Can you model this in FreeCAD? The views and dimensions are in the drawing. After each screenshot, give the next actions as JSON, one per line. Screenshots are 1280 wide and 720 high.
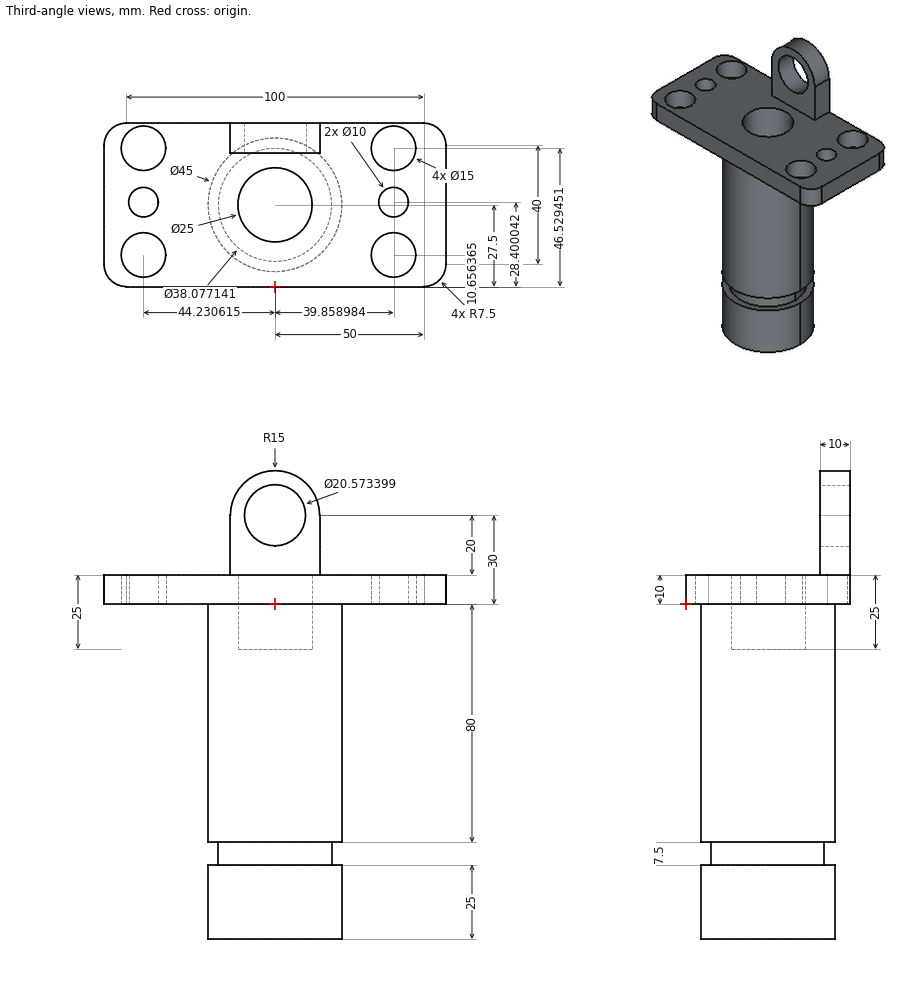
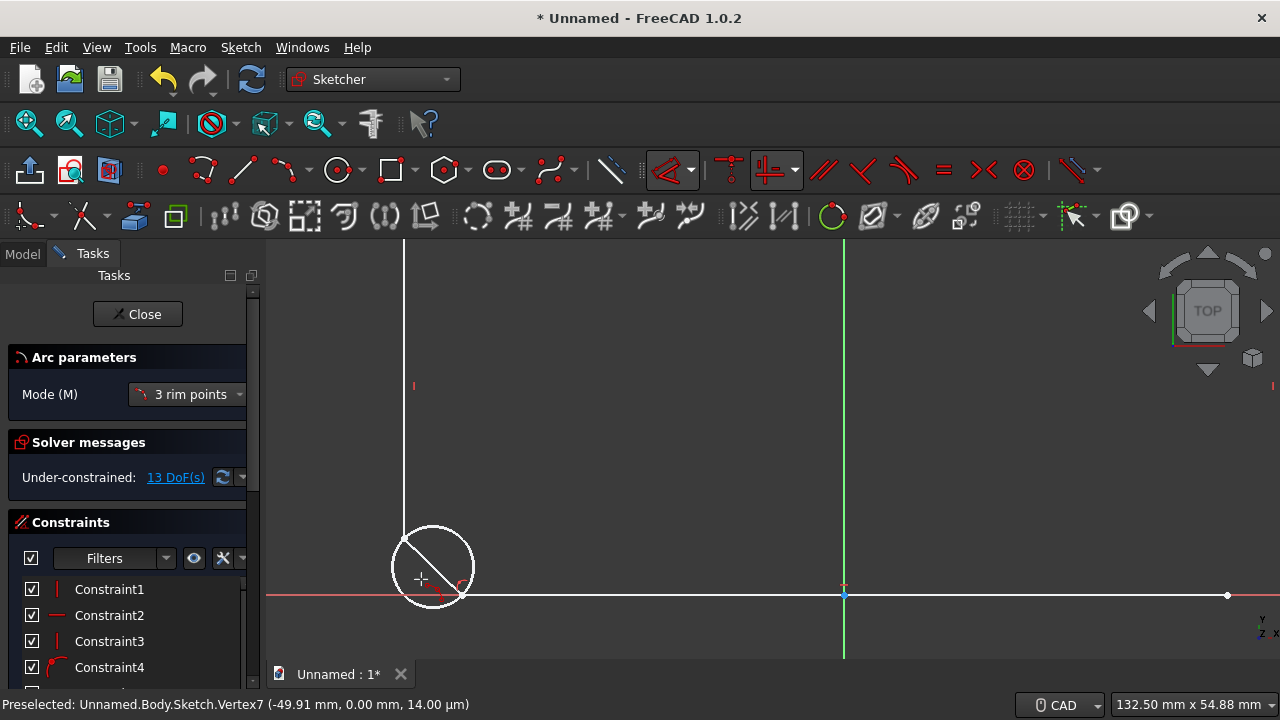
{"action": "left_click", "coordinate": [421, 579]}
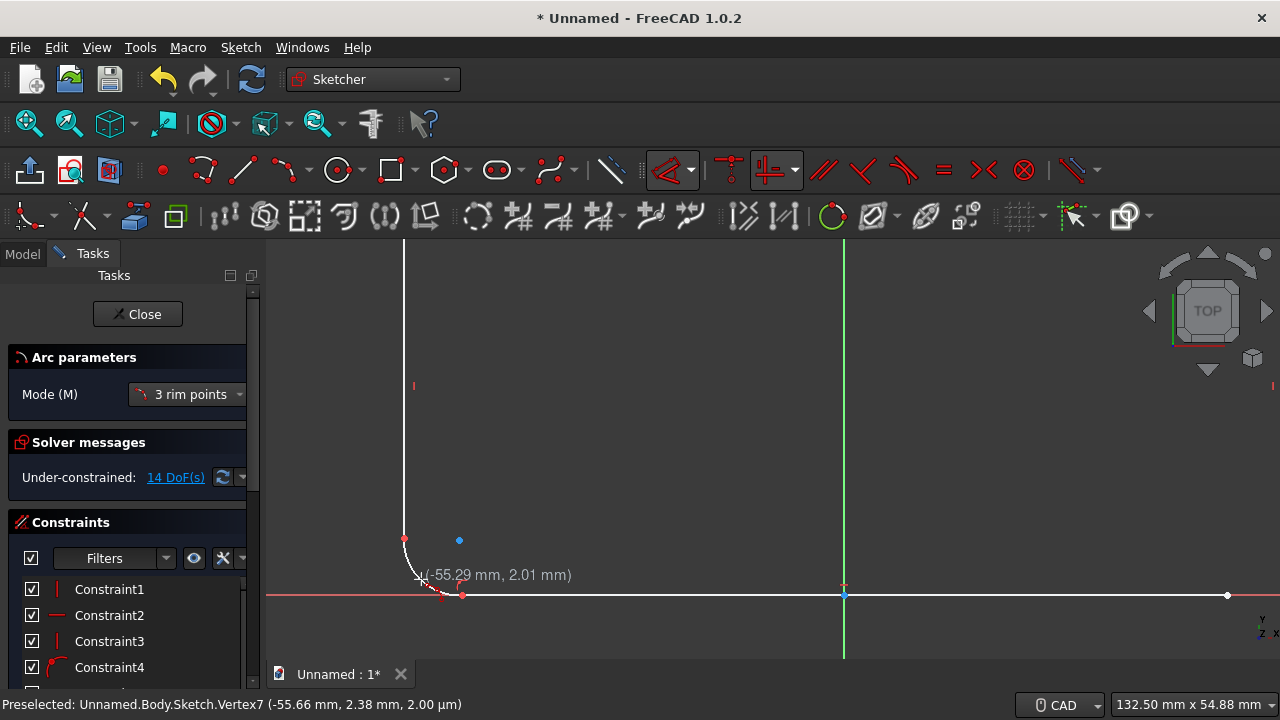
{"action": "scroll", "coordinate": [421, 579], "scroll_direction": "down", "scroll_amount": 2}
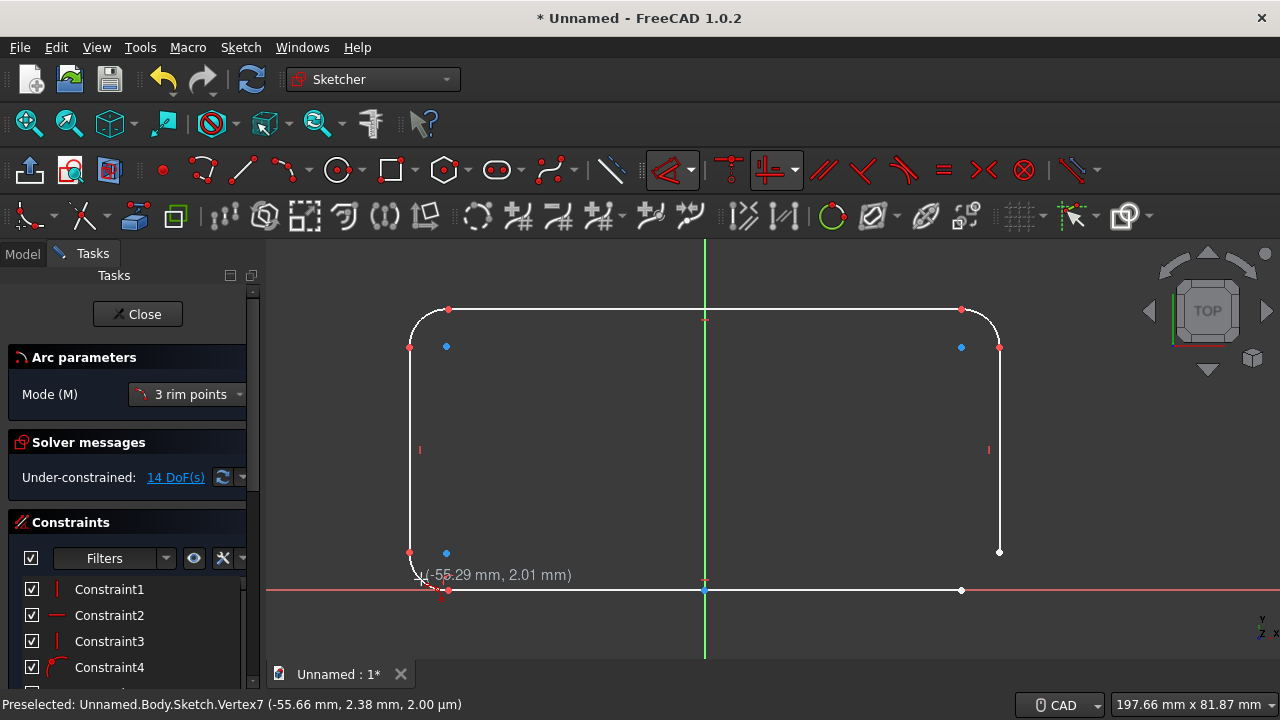
{"action": "left_click", "coordinate": [962, 590]}
{"action": "left_click", "coordinate": [1000, 552]}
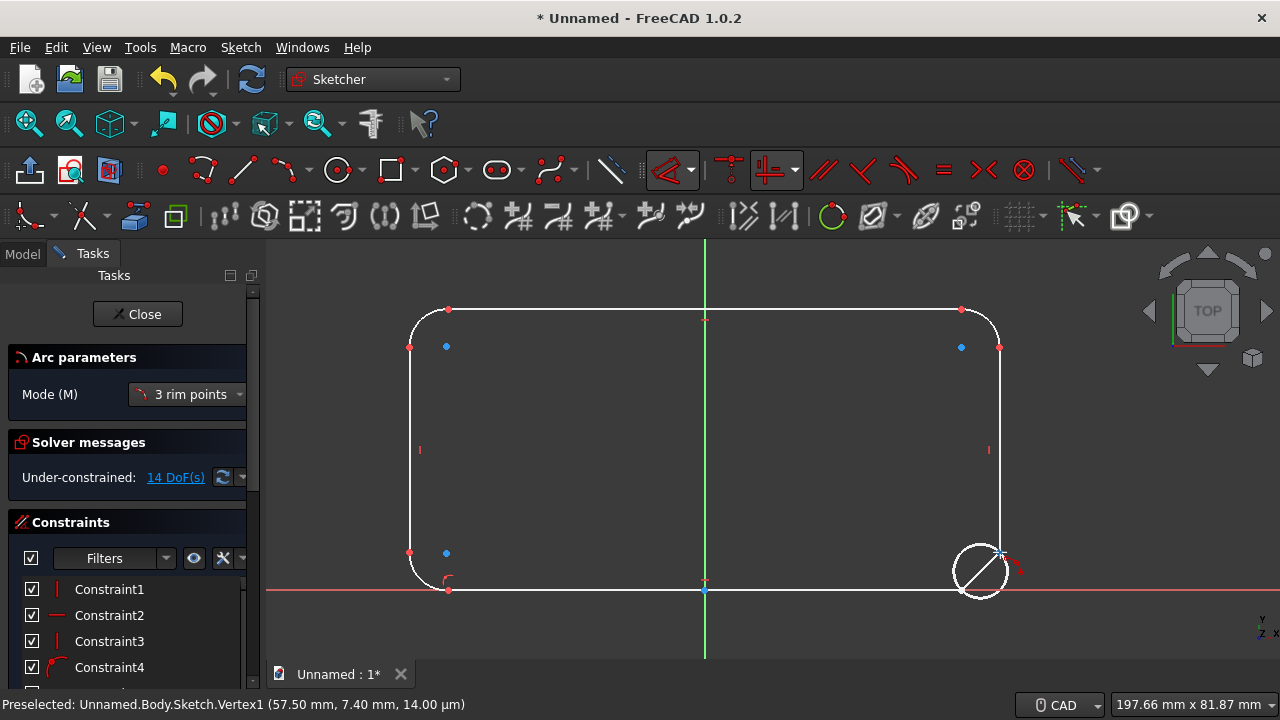
{"action": "scroll", "coordinate": [988, 579], "scroll_direction": "up", "scroll_amount": 2}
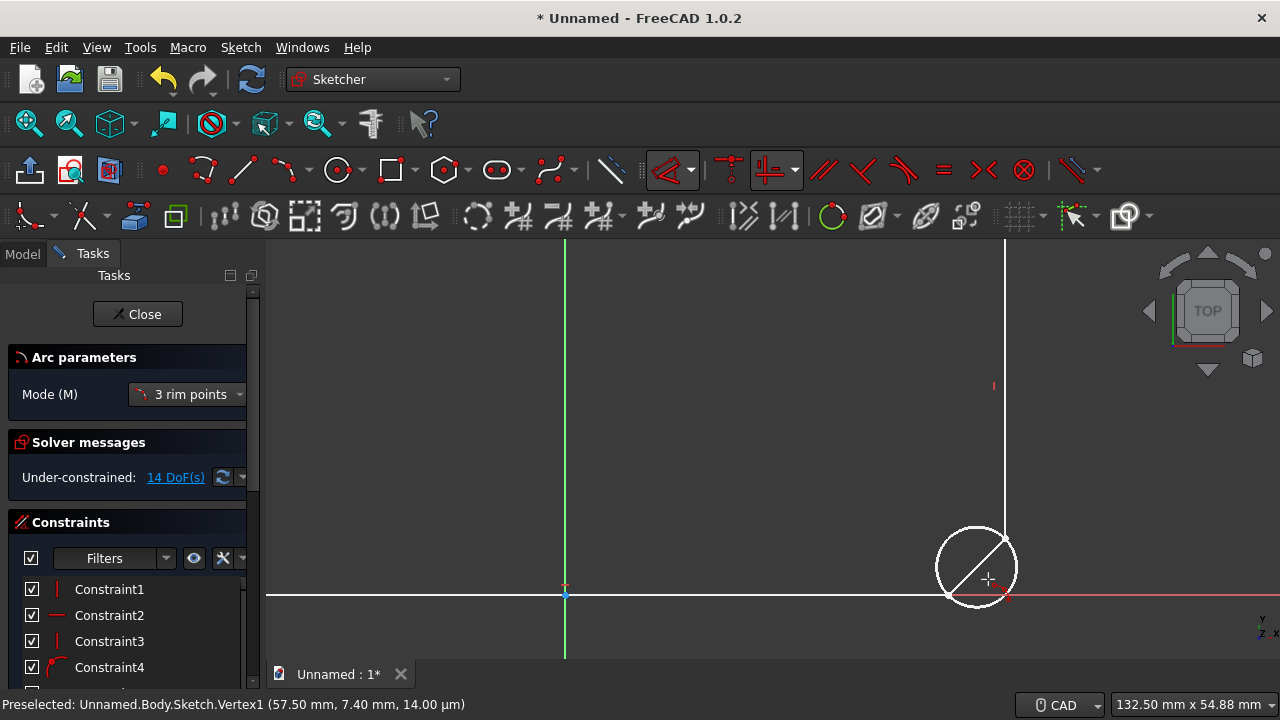
{"action": "left_click", "coordinate": [988, 579]}
{"action": "key", "text": "Escape"}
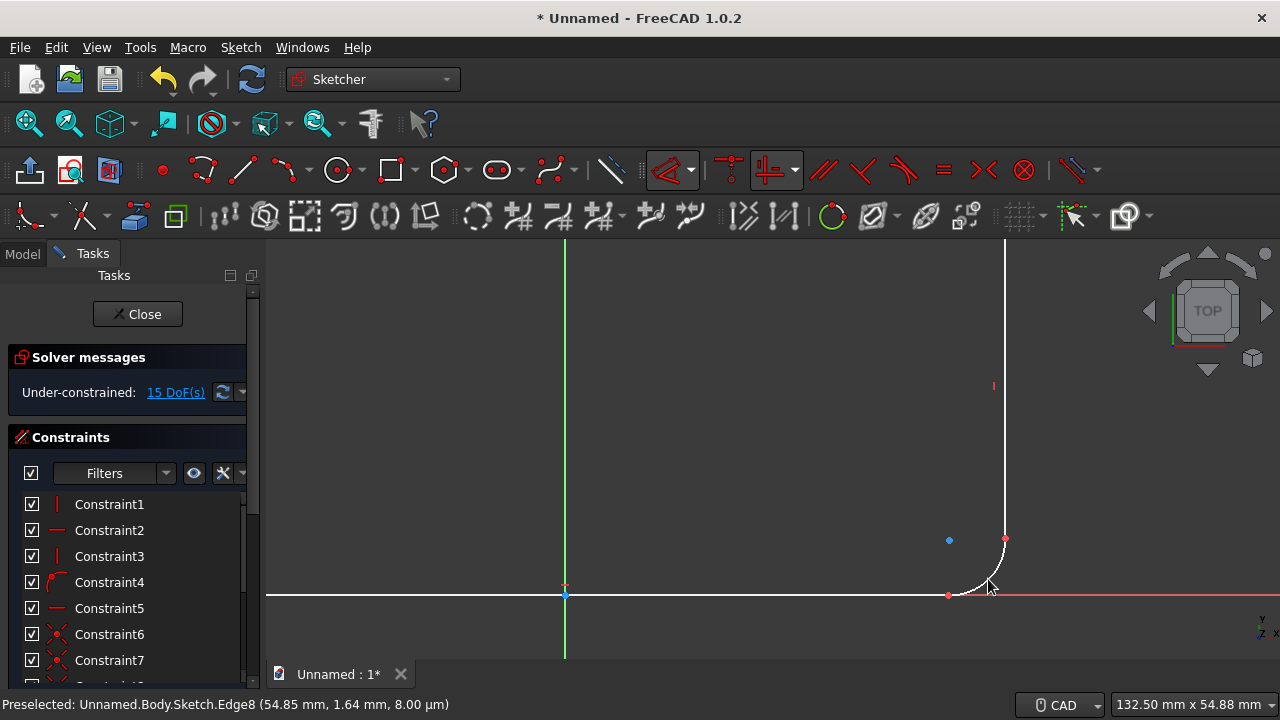
{"action": "left_click", "coordinate": [1005, 447]}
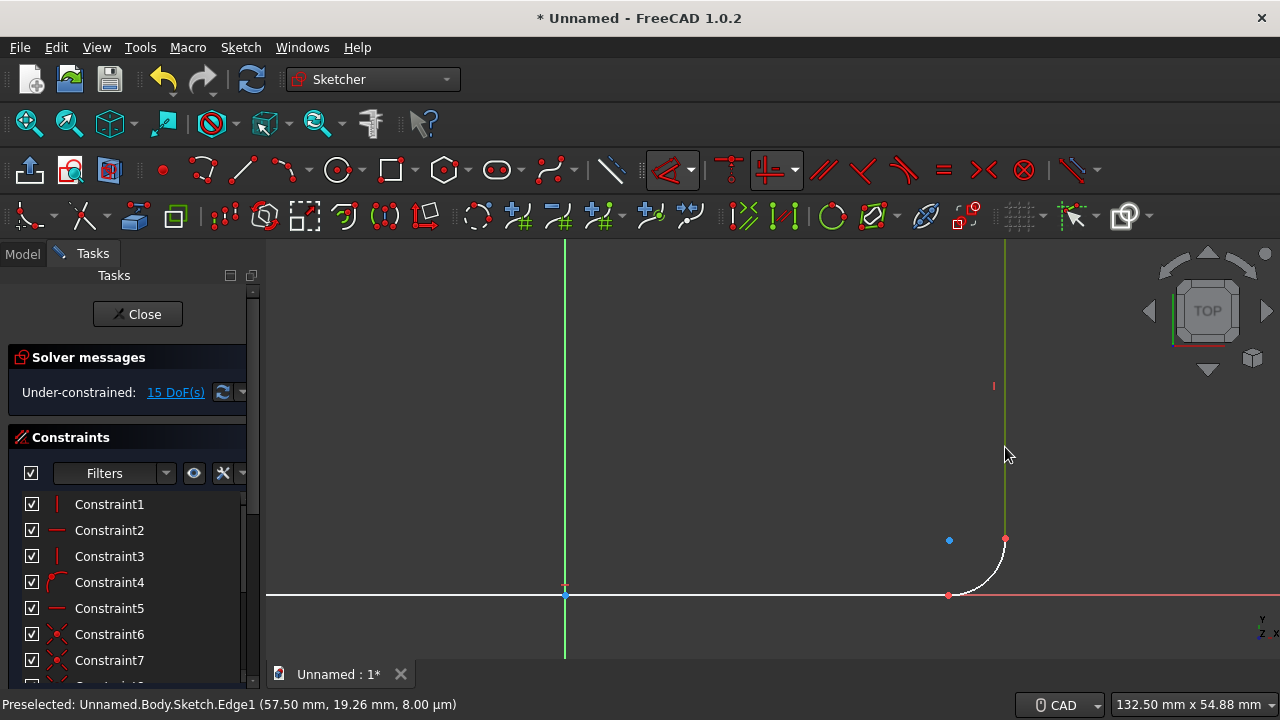
{"action": "scroll", "coordinate": [988, 579], "scroll_direction": "down", "scroll_amount": 2}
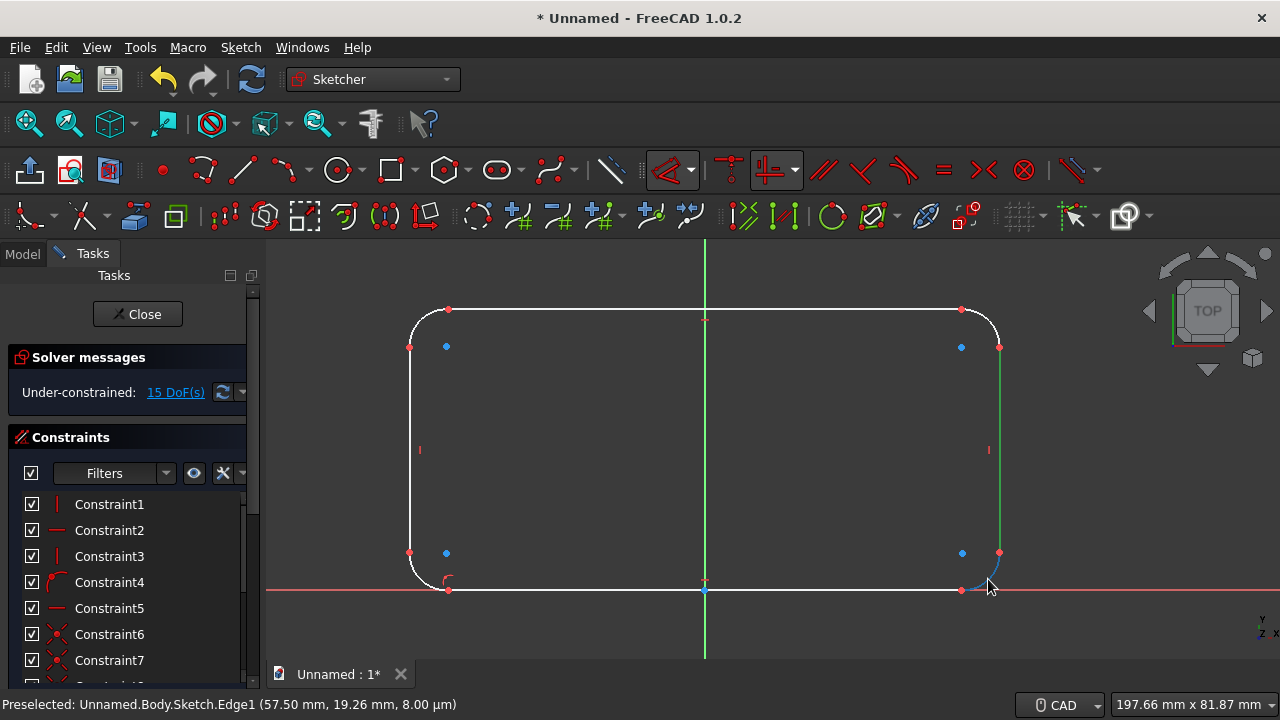
{"action": "left_click", "coordinate": [996, 330]}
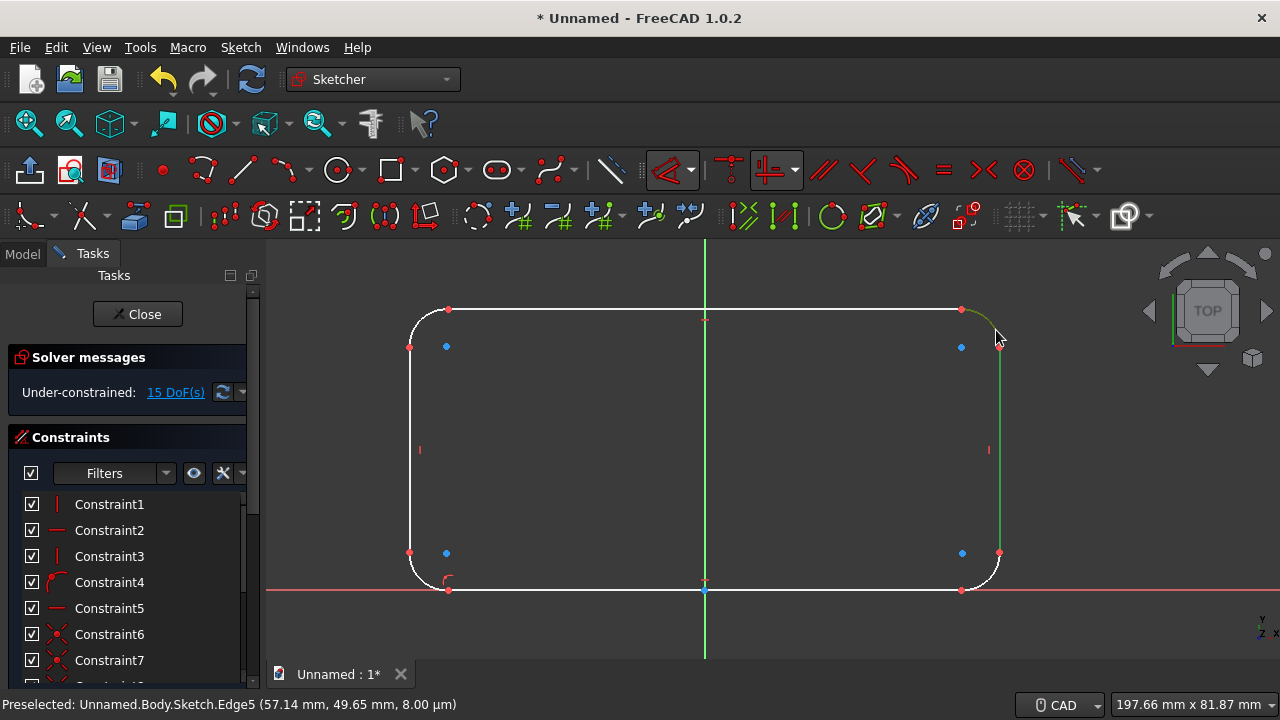
{"action": "left_click", "coordinate": [904, 170]}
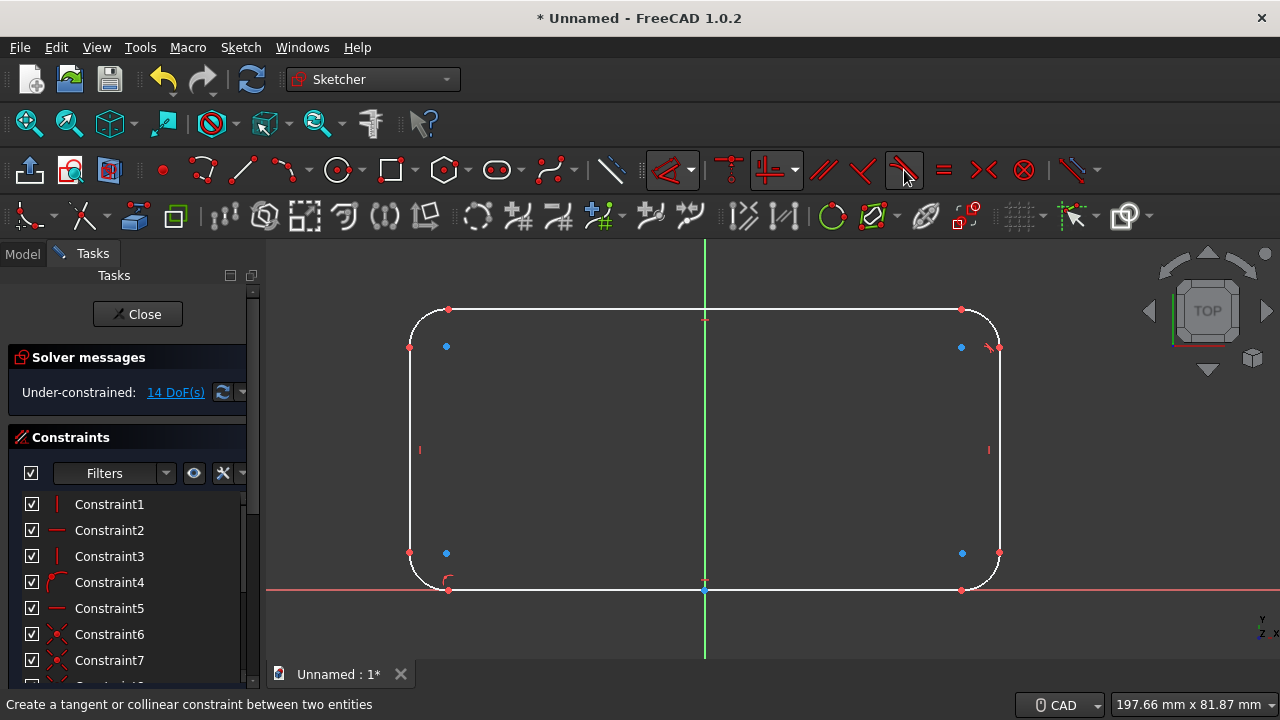
{"action": "left_click", "coordinate": [1000, 491]}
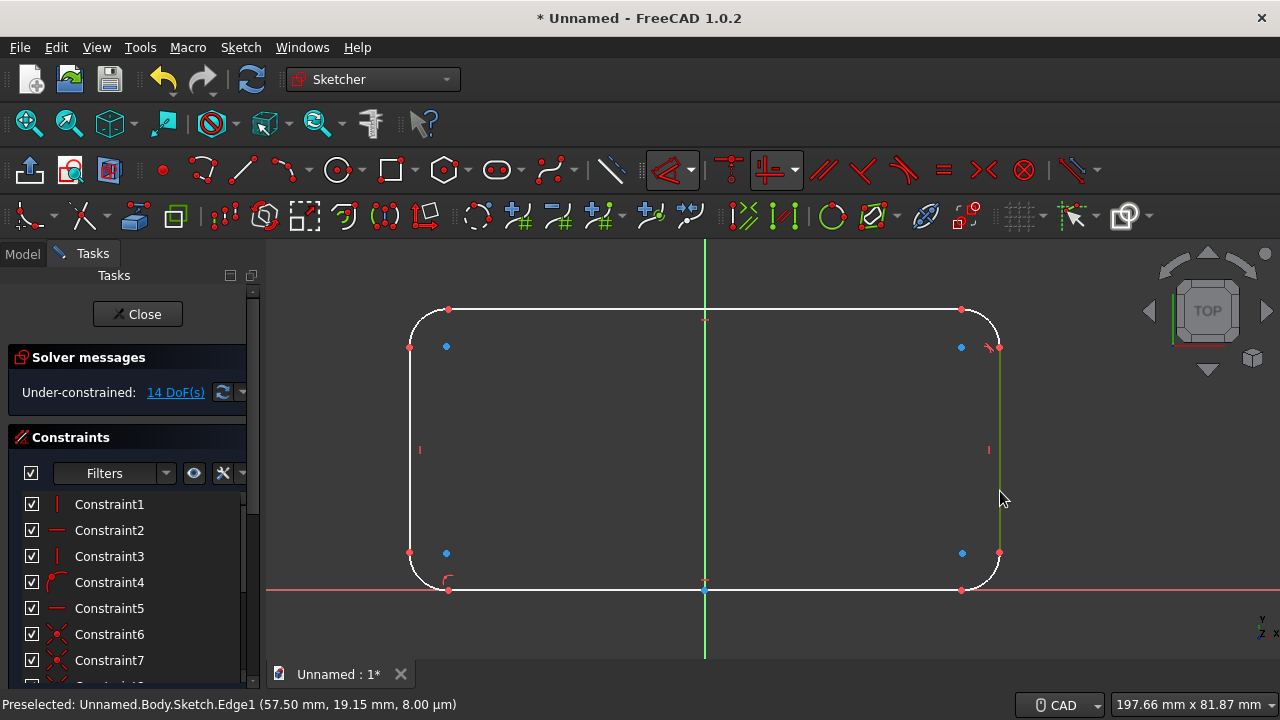
{"action": "left_click", "coordinate": [979, 586]}